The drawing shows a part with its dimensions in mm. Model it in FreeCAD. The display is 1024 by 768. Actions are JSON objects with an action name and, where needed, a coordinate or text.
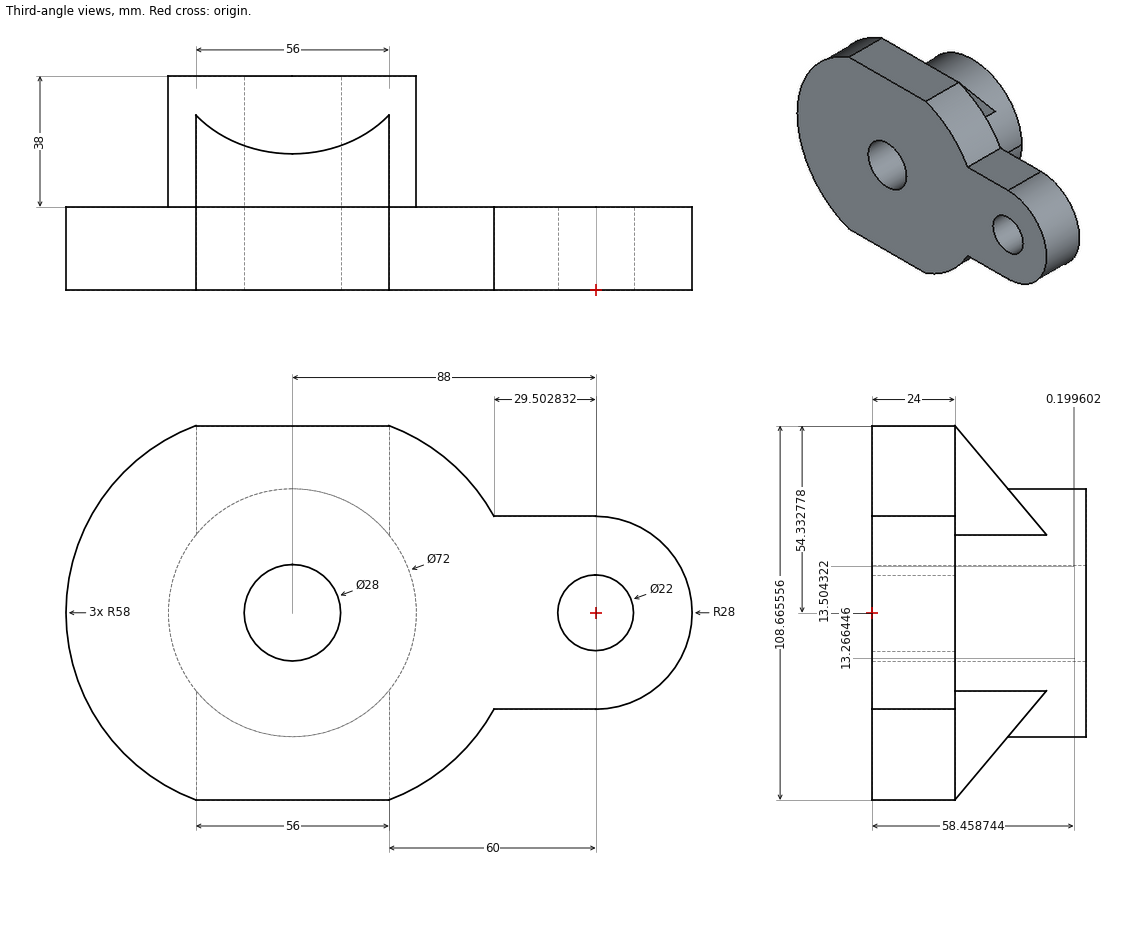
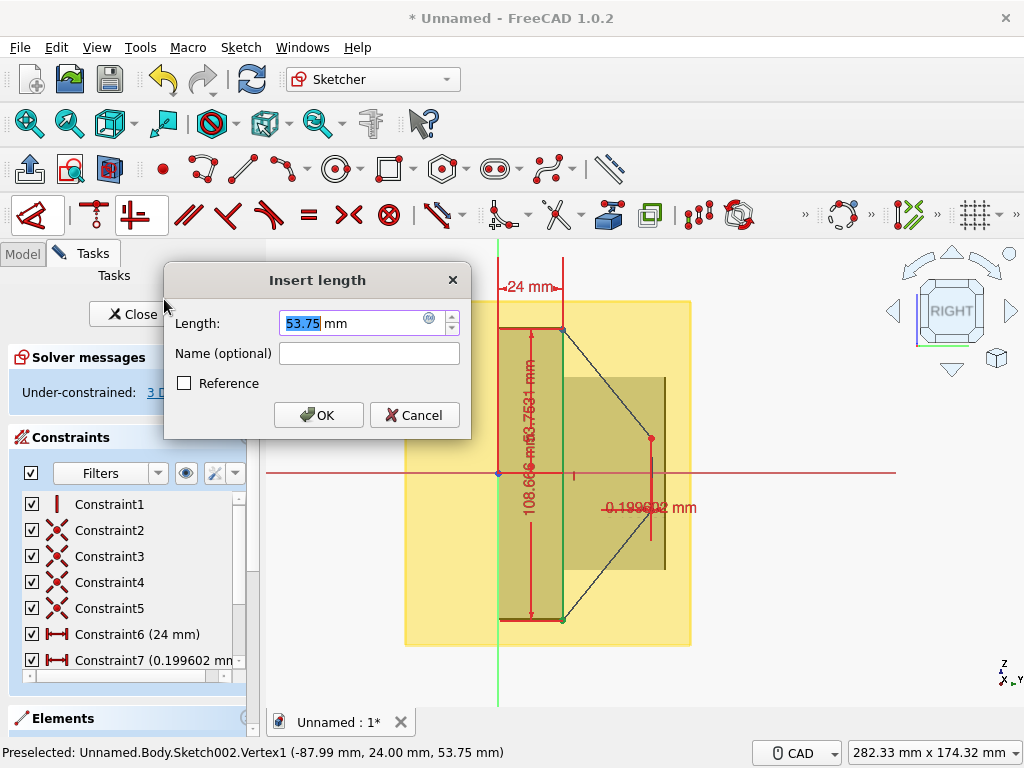
{"action": "type", "text": "54.332778"}
{"action": "key", "text": "Return"}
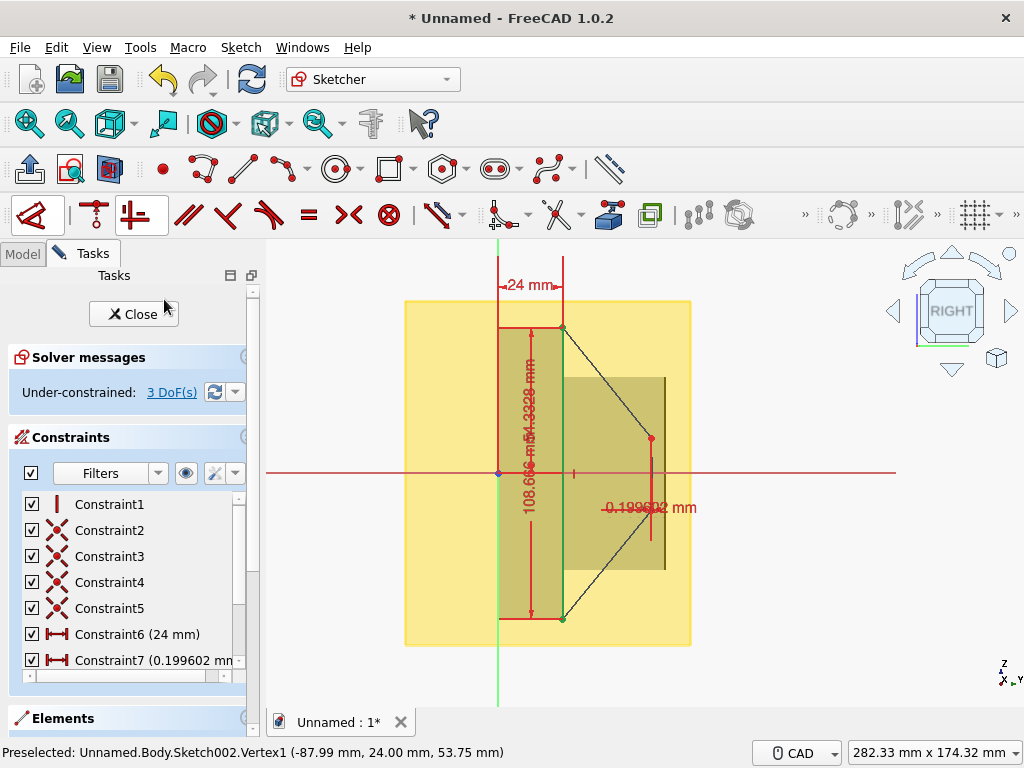
{"action": "left_click", "coordinate": [652, 510]}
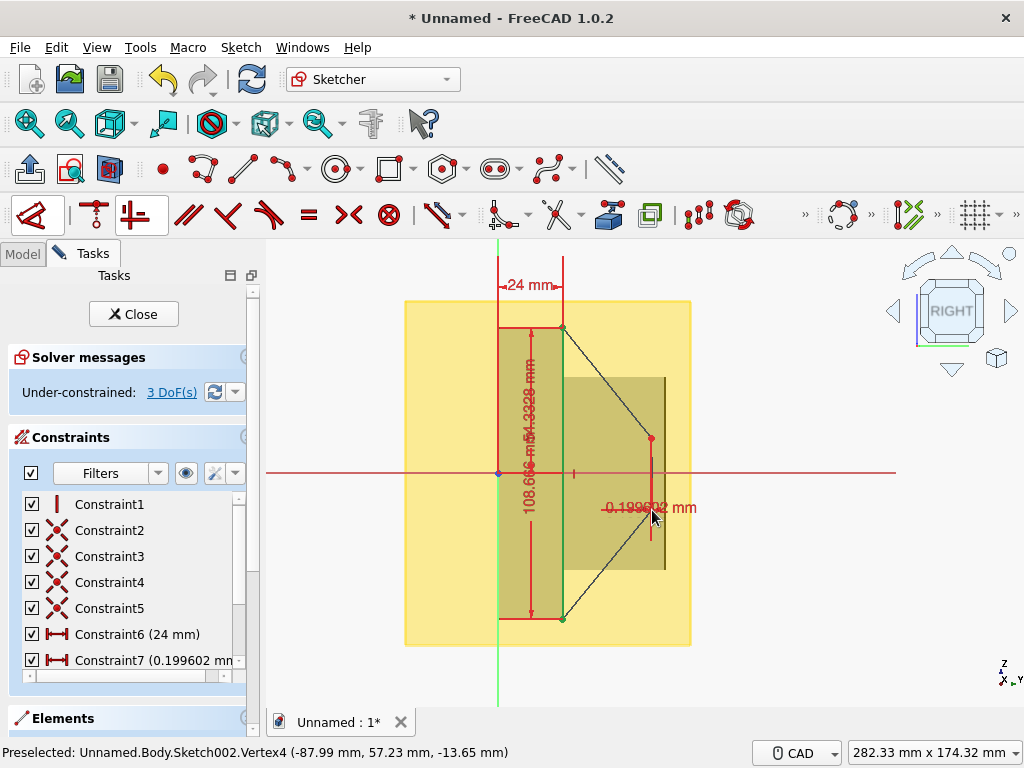
{"action": "key", "text": "l"}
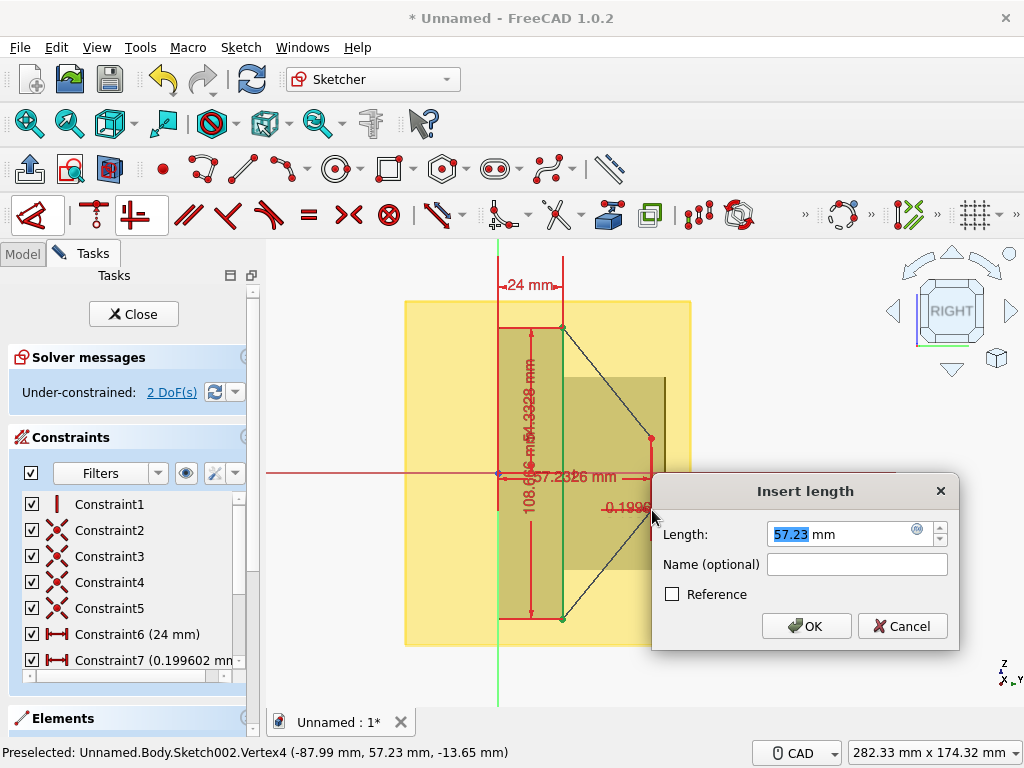
{"action": "type", "text": "58.458744"}
{"action": "key", "text": "Return"}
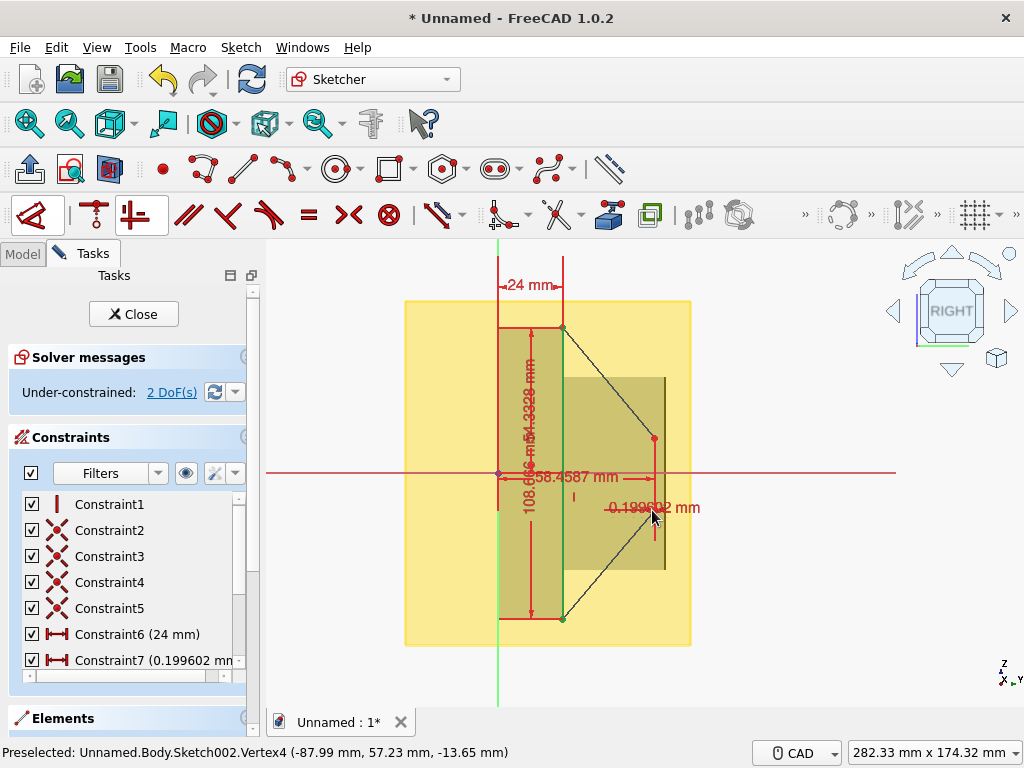
{"action": "left_click", "coordinate": [655, 510]}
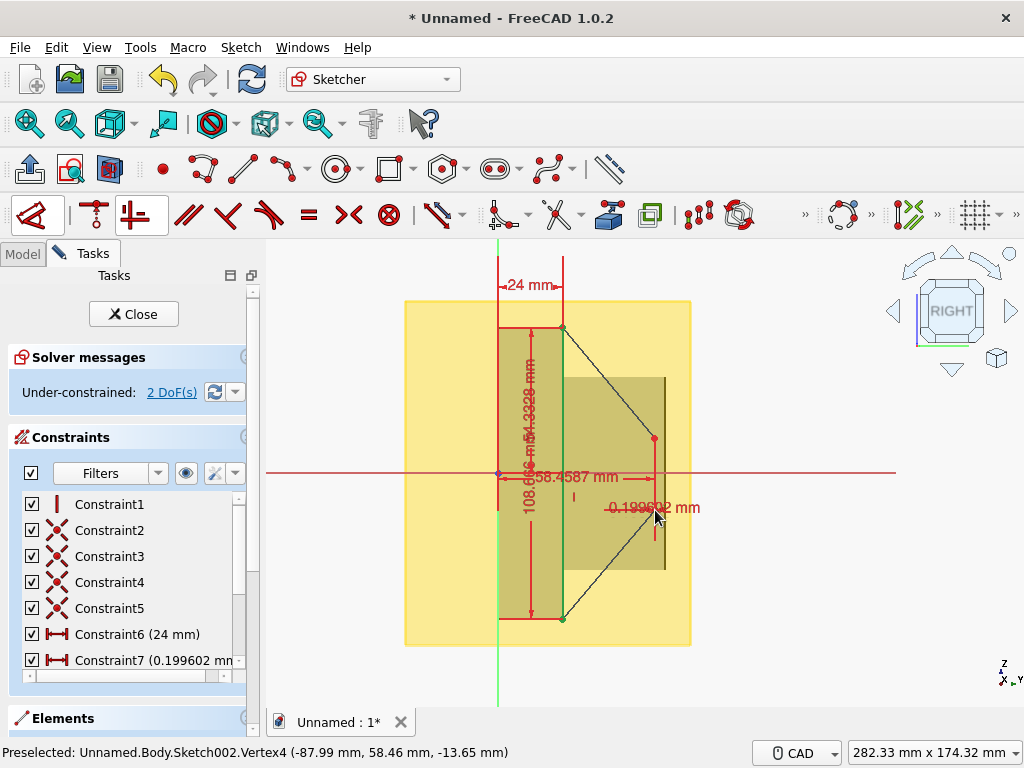
{"action": "left_click", "coordinate": [58, 216]}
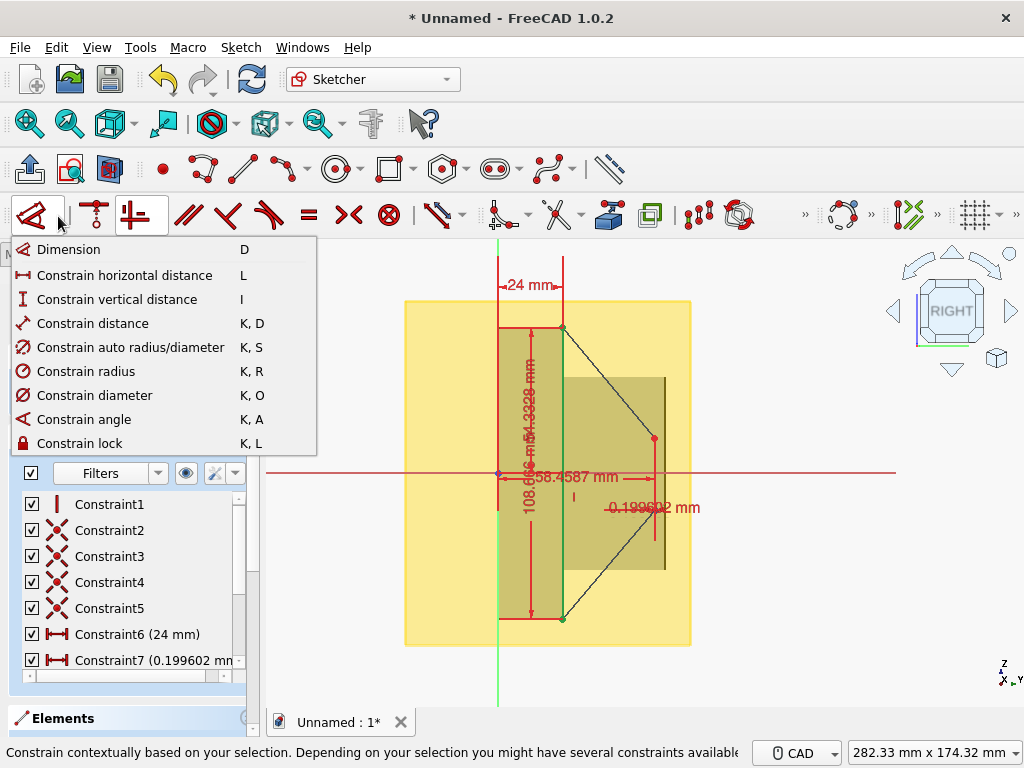
{"action": "left_click", "coordinate": [164, 299]}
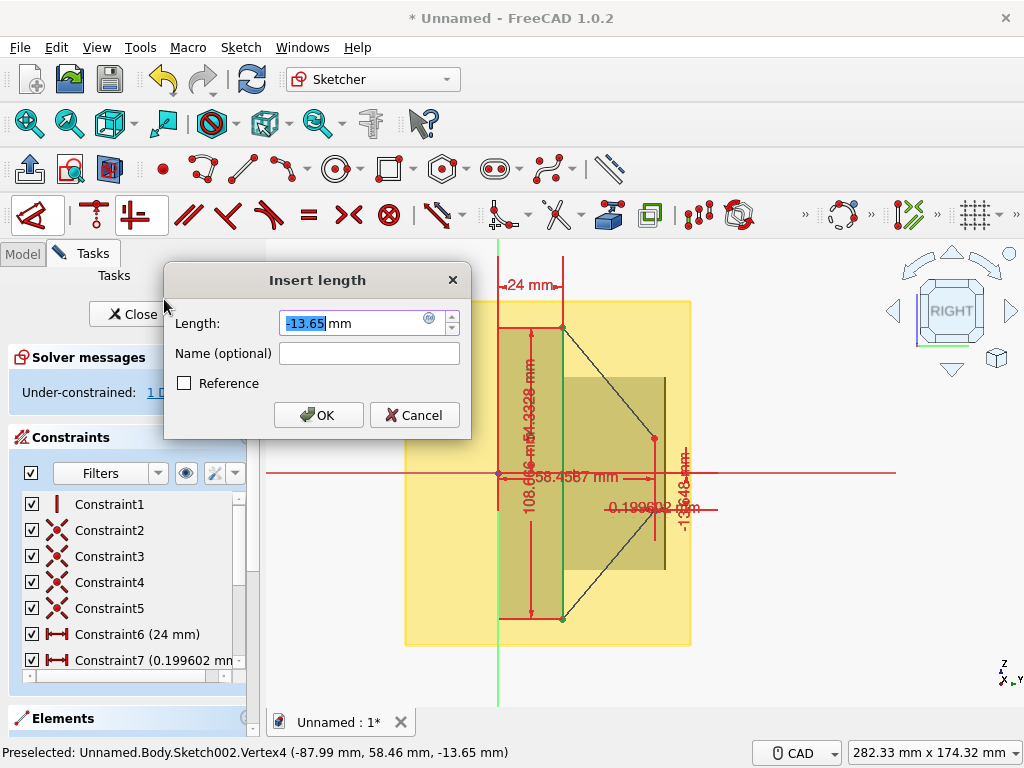
{"action": "type", "text": "-13.266446"}
{"action": "key", "text": "Return"}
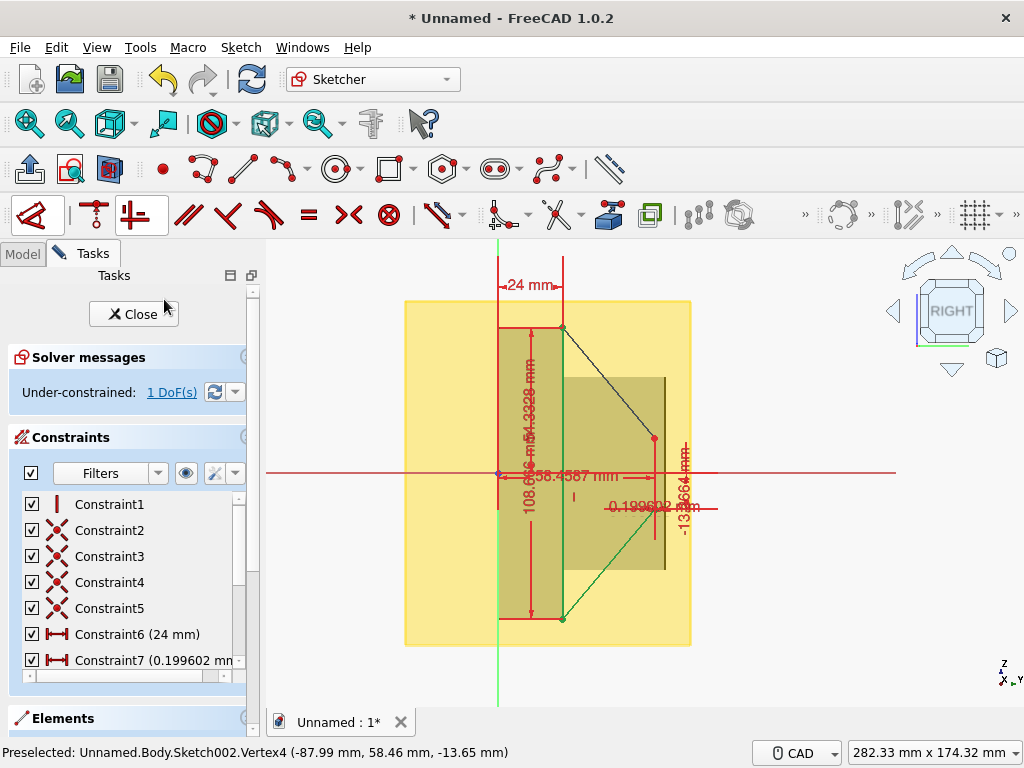
{"action": "left_click", "coordinate": [655, 438]}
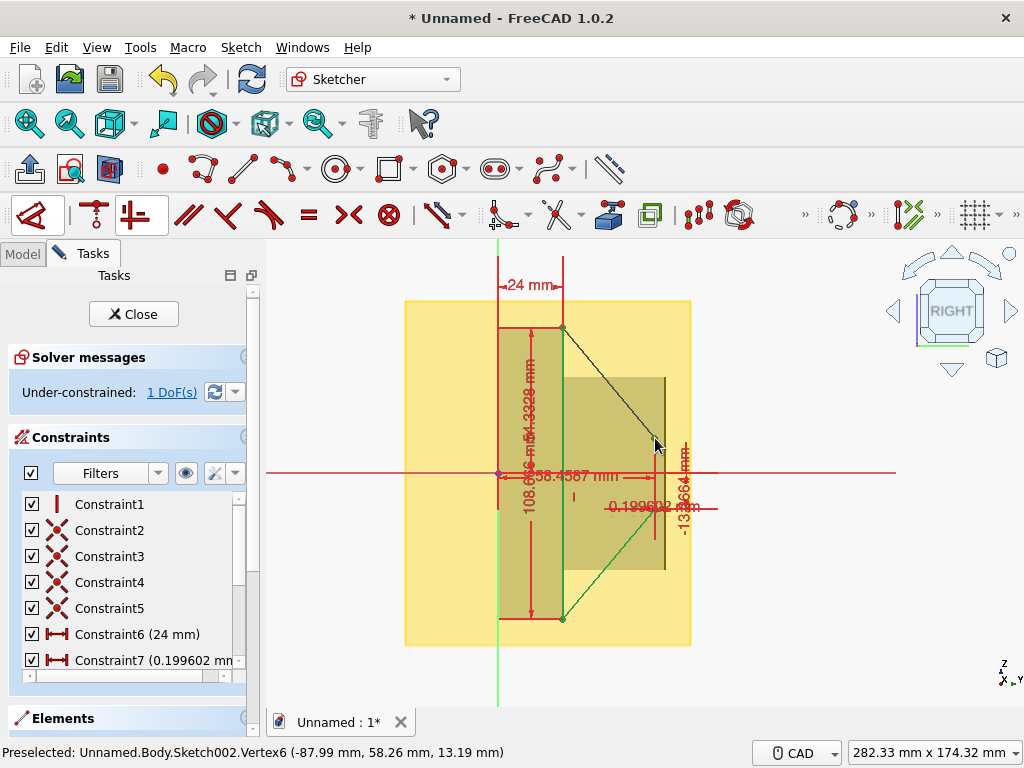
{"action": "left_click", "coordinate": [58, 216]}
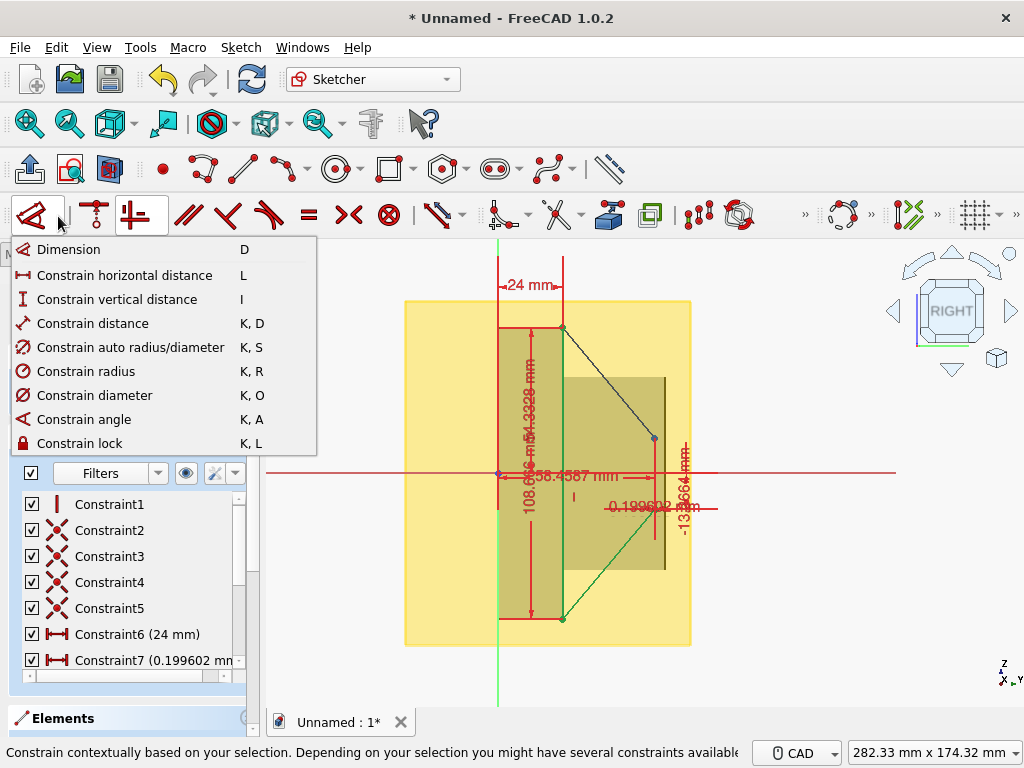
{"action": "left_click", "coordinate": [164, 299]}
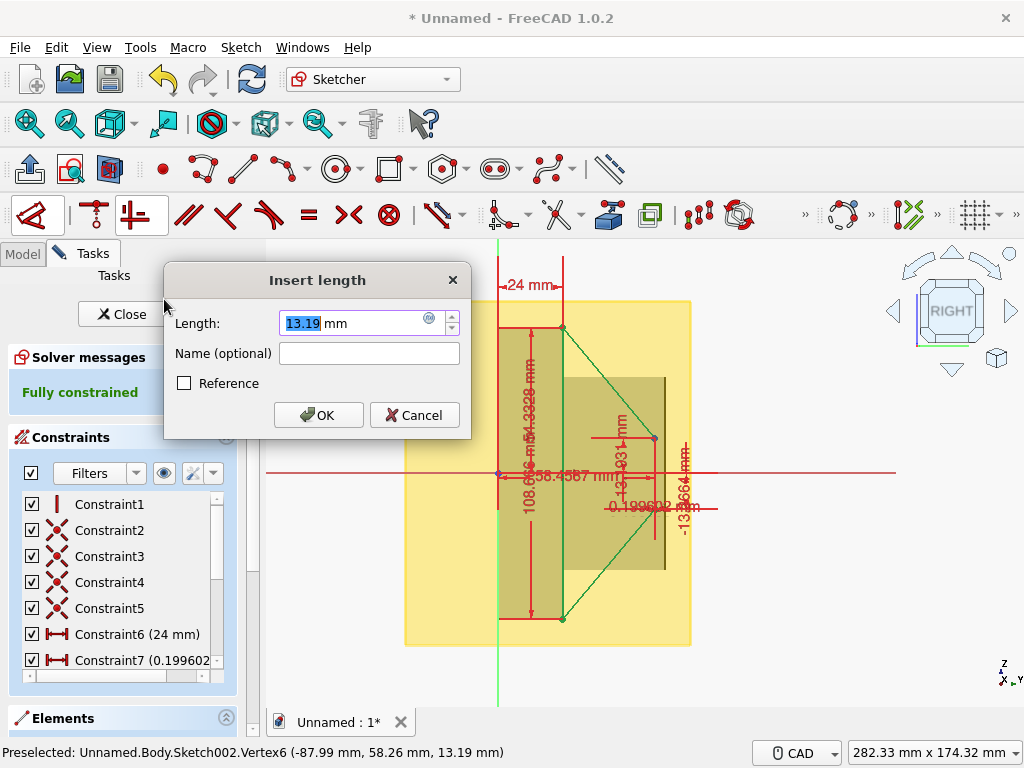
{"action": "type", "text": "13.504322"}
{"action": "key", "text": "Return"}